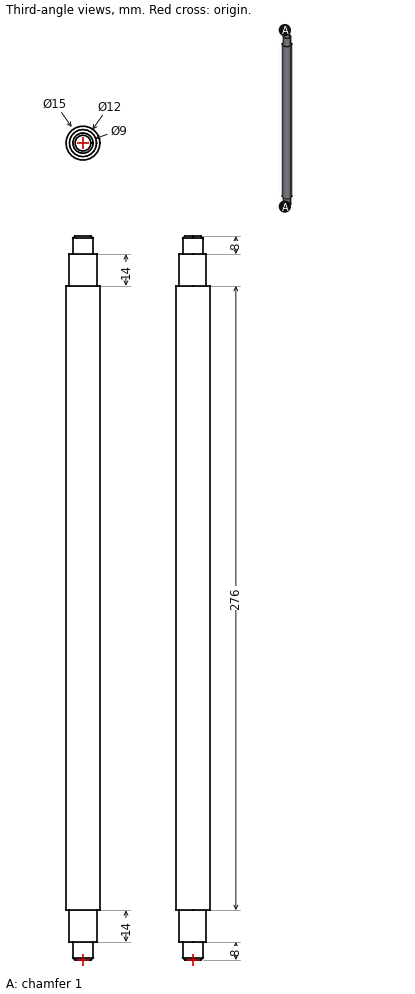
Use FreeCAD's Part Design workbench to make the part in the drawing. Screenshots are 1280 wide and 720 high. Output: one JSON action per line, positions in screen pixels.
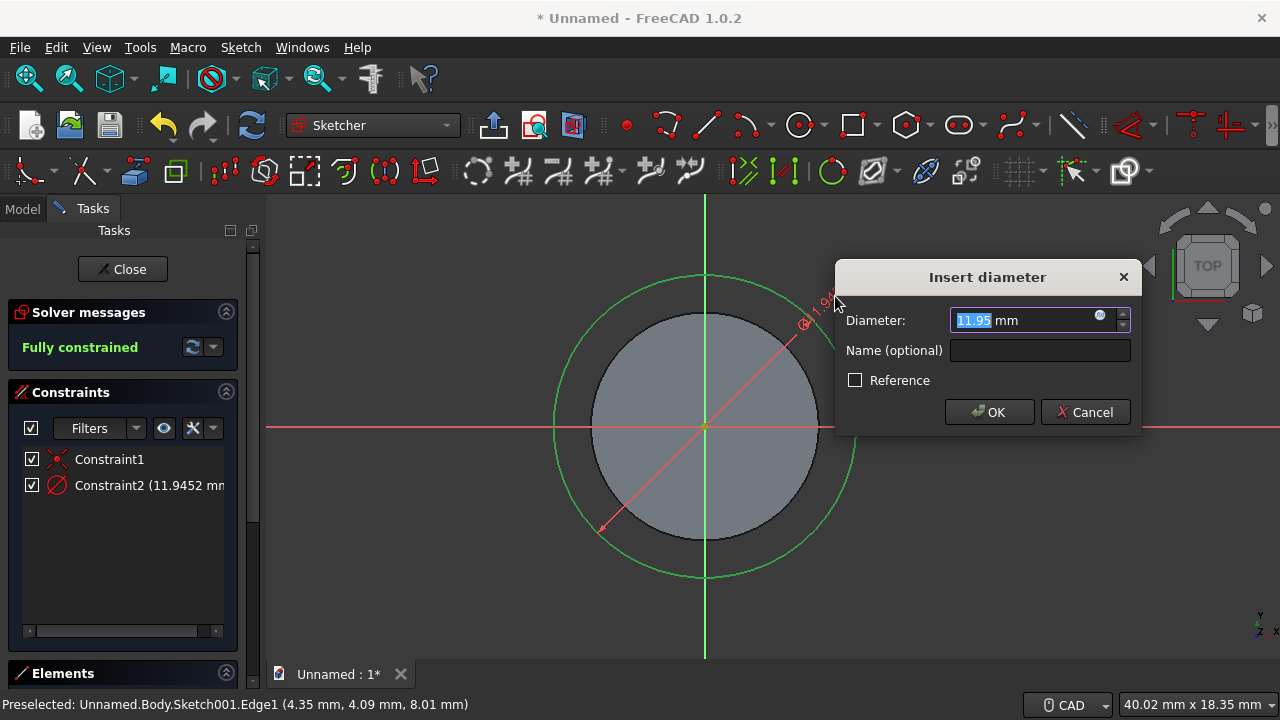
{"action": "type", "text": "12"}
{"action": "key", "text": "Return"}
{"action": "key", "text": "Escape"}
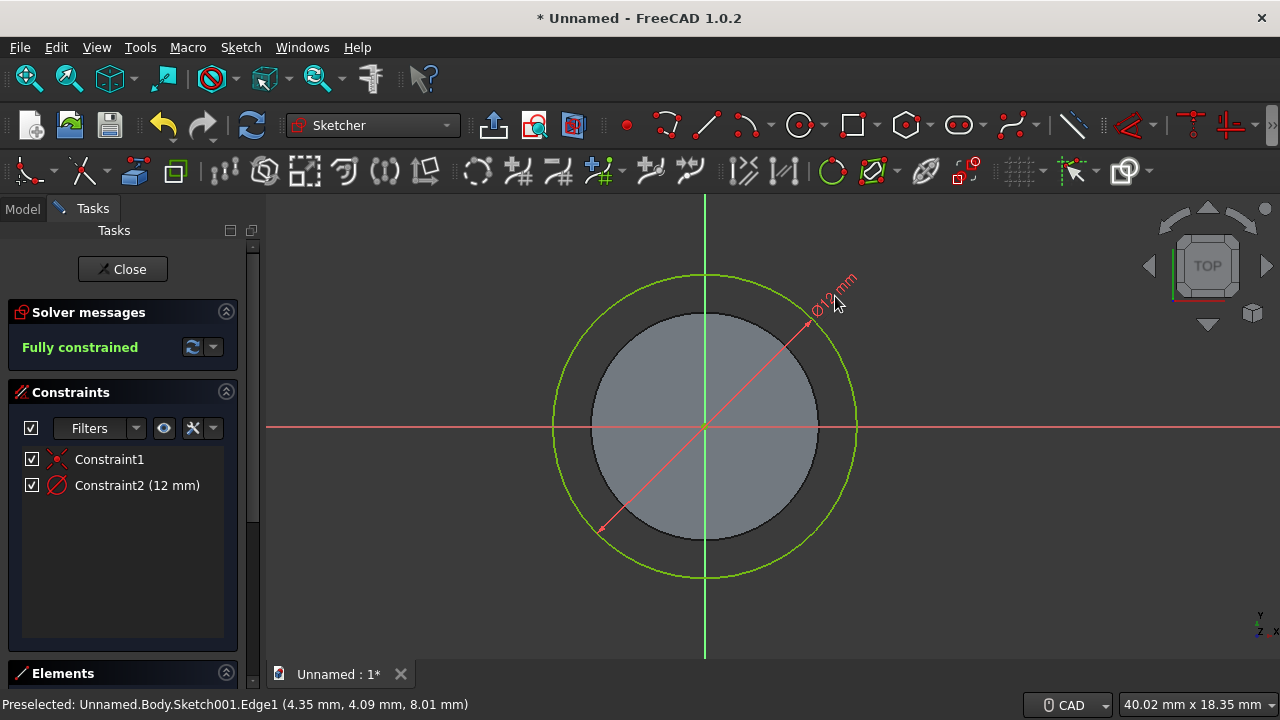
{"action": "left_click", "coordinate": [123, 269]}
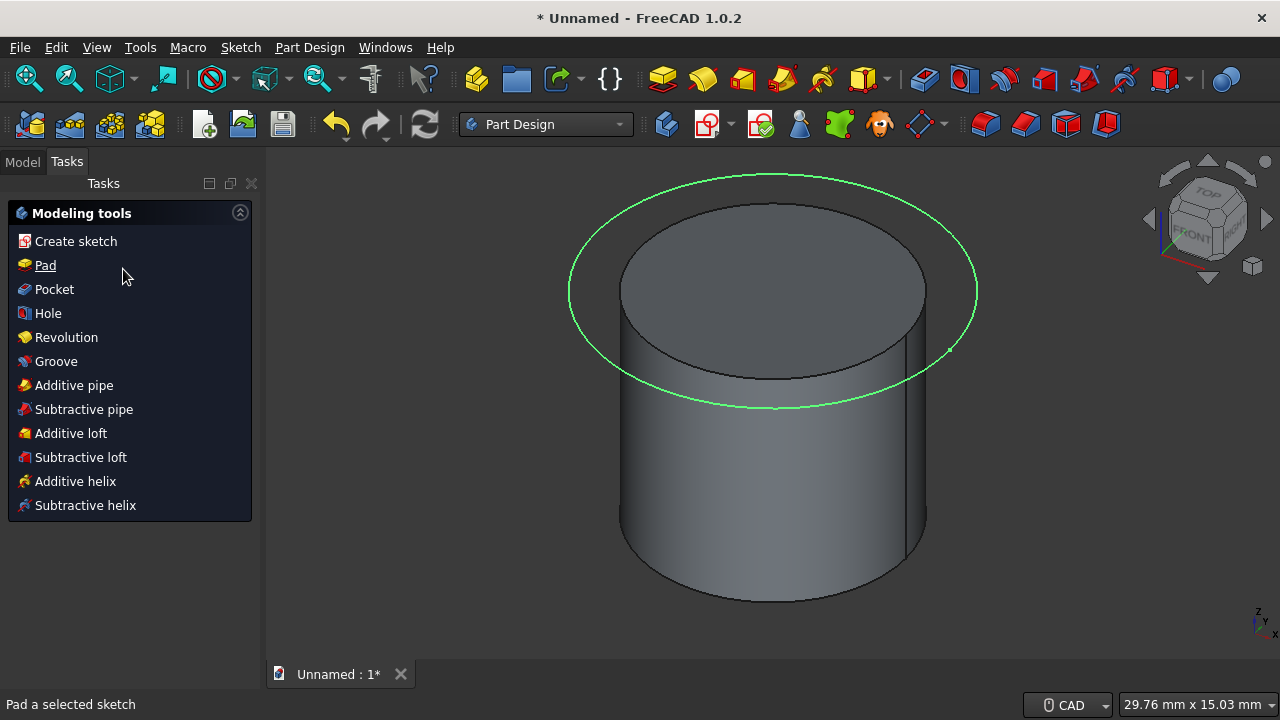
{"action": "left_click", "coordinate": [664, 80]}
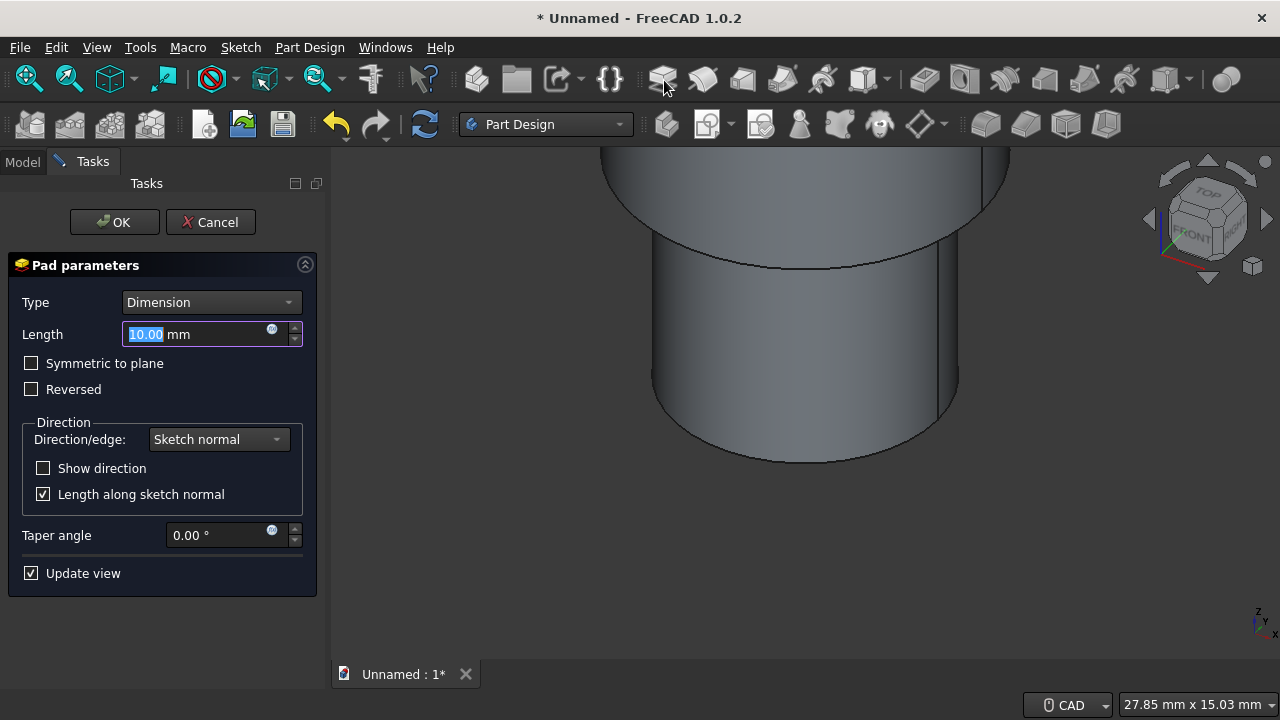
{"action": "type", "text": "14"}
{"action": "key", "text": "Tab"}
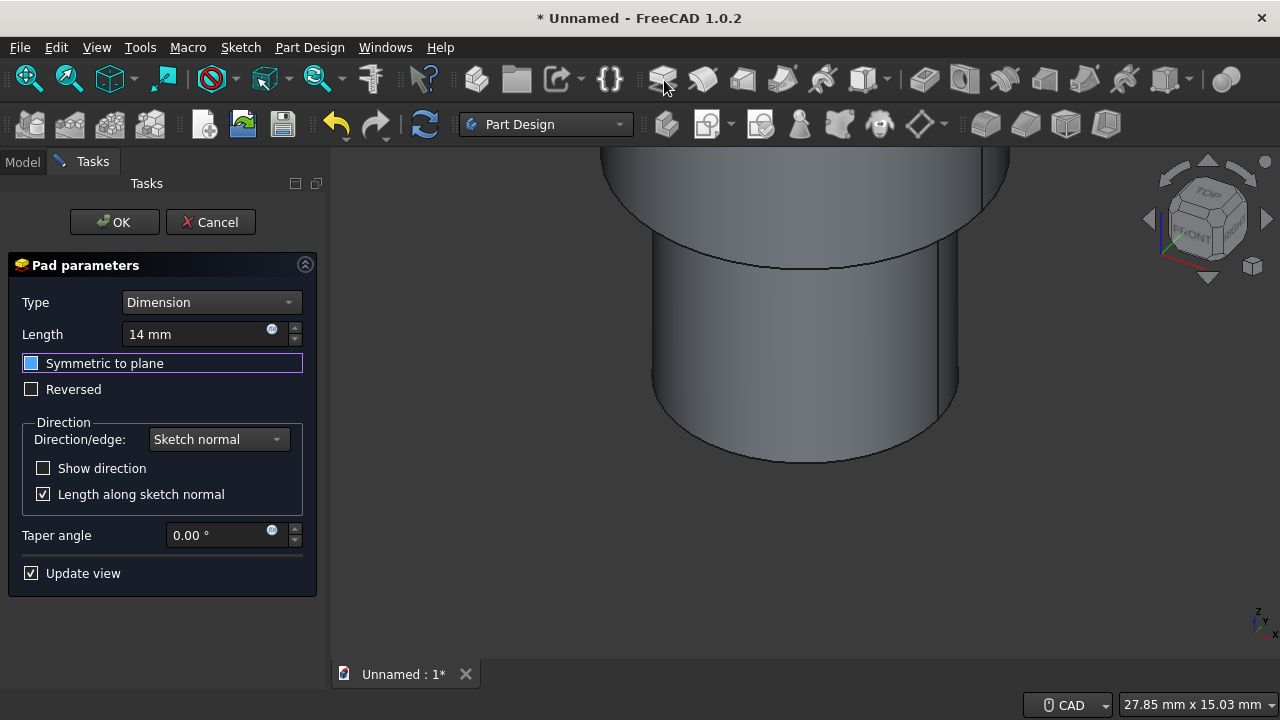
{"action": "left_click", "coordinate": [115, 222]}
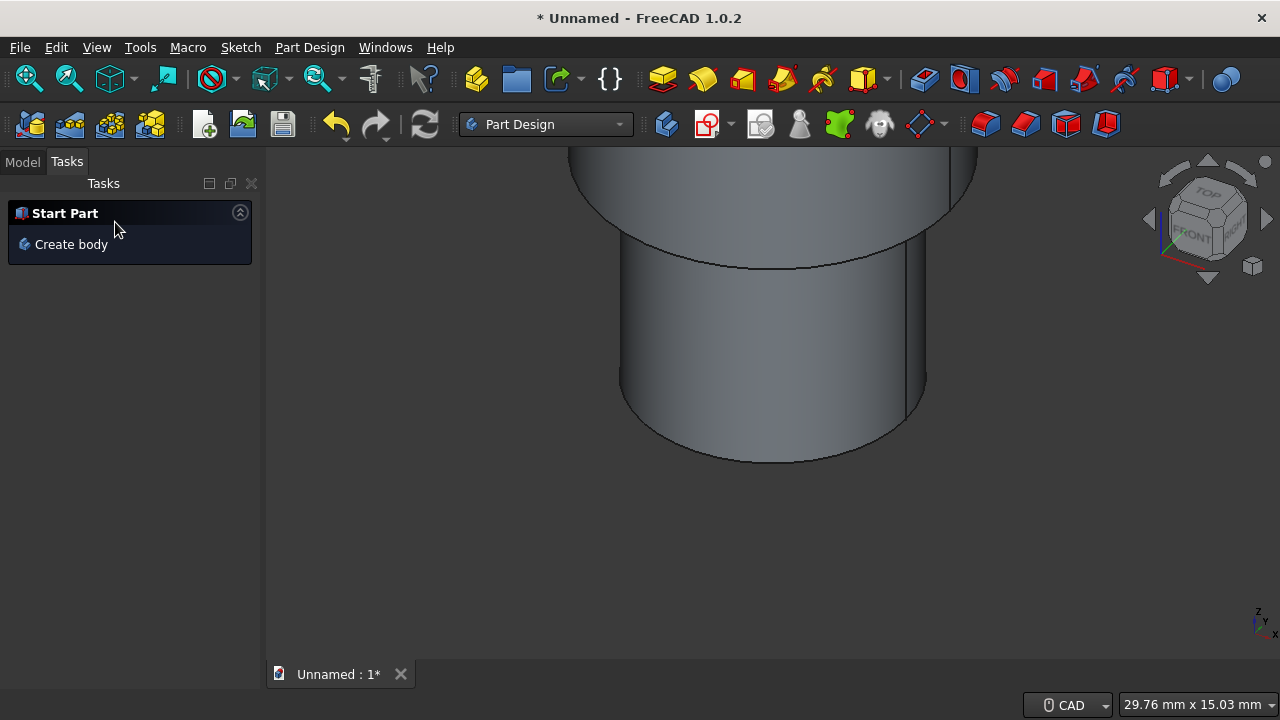
{"action": "left_click", "coordinate": [30, 80]}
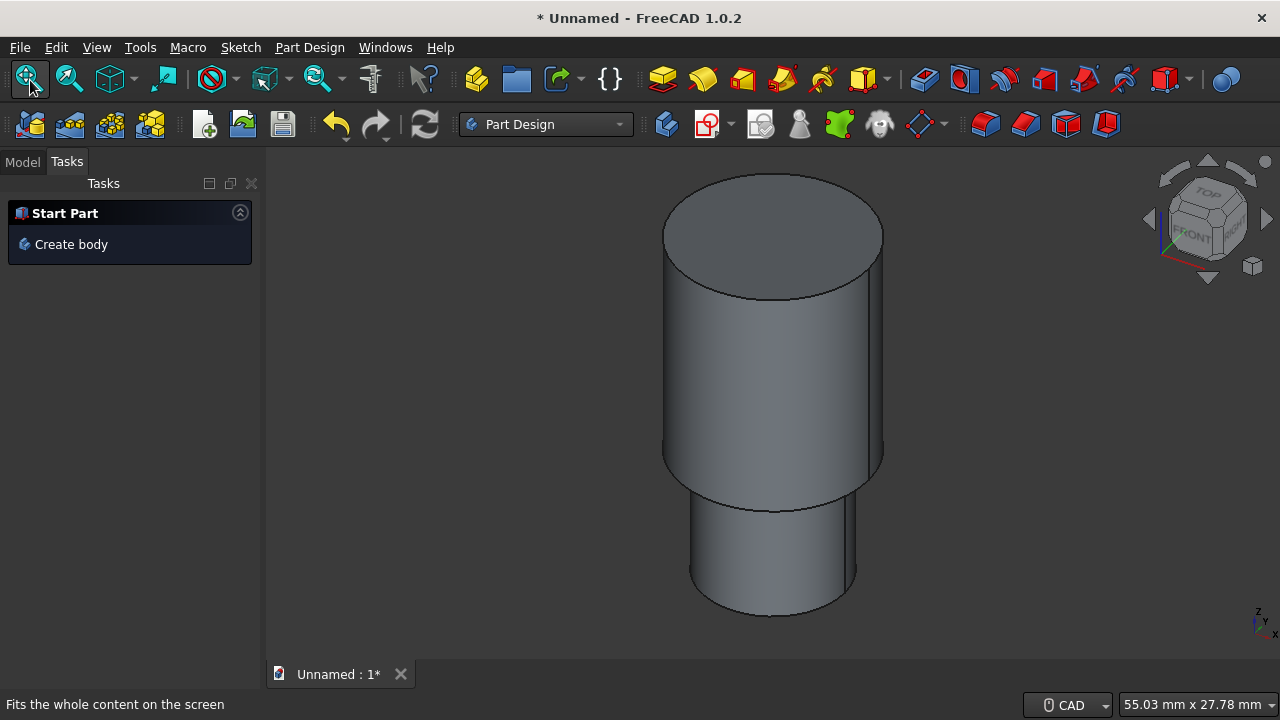
{"action": "left_click", "coordinate": [773, 236]}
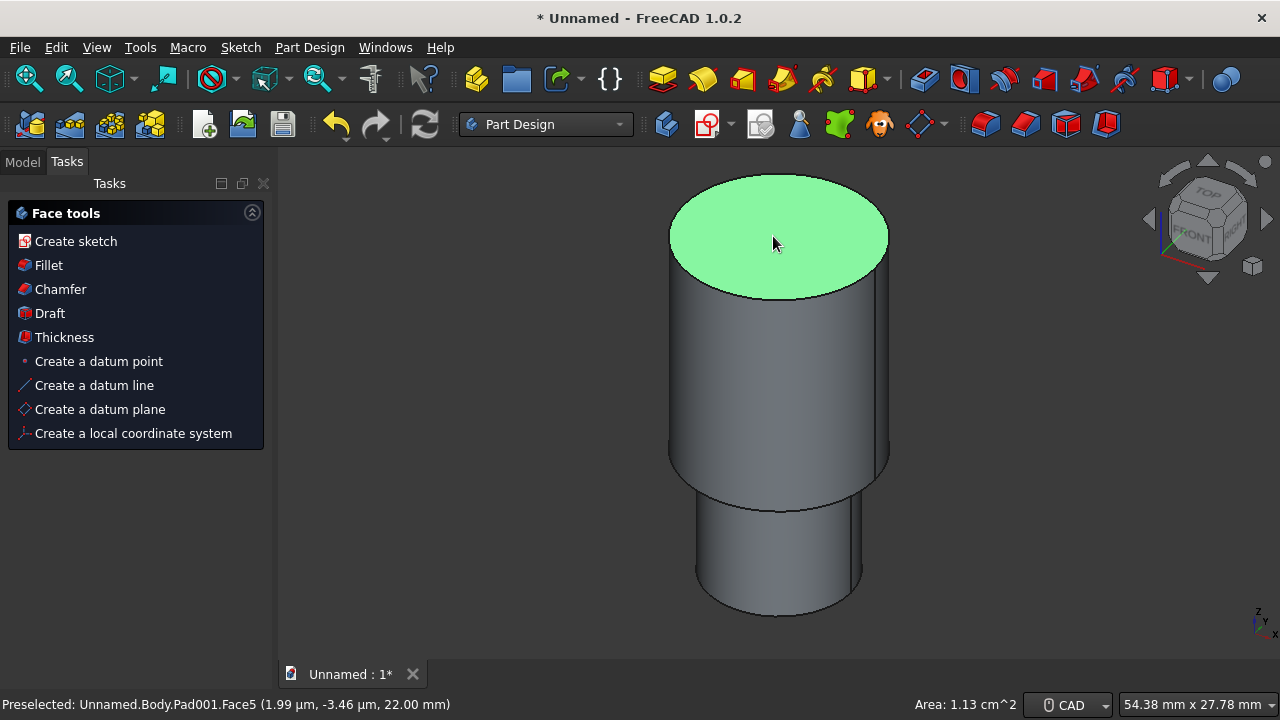
{"action": "left_click", "coordinate": [708, 124]}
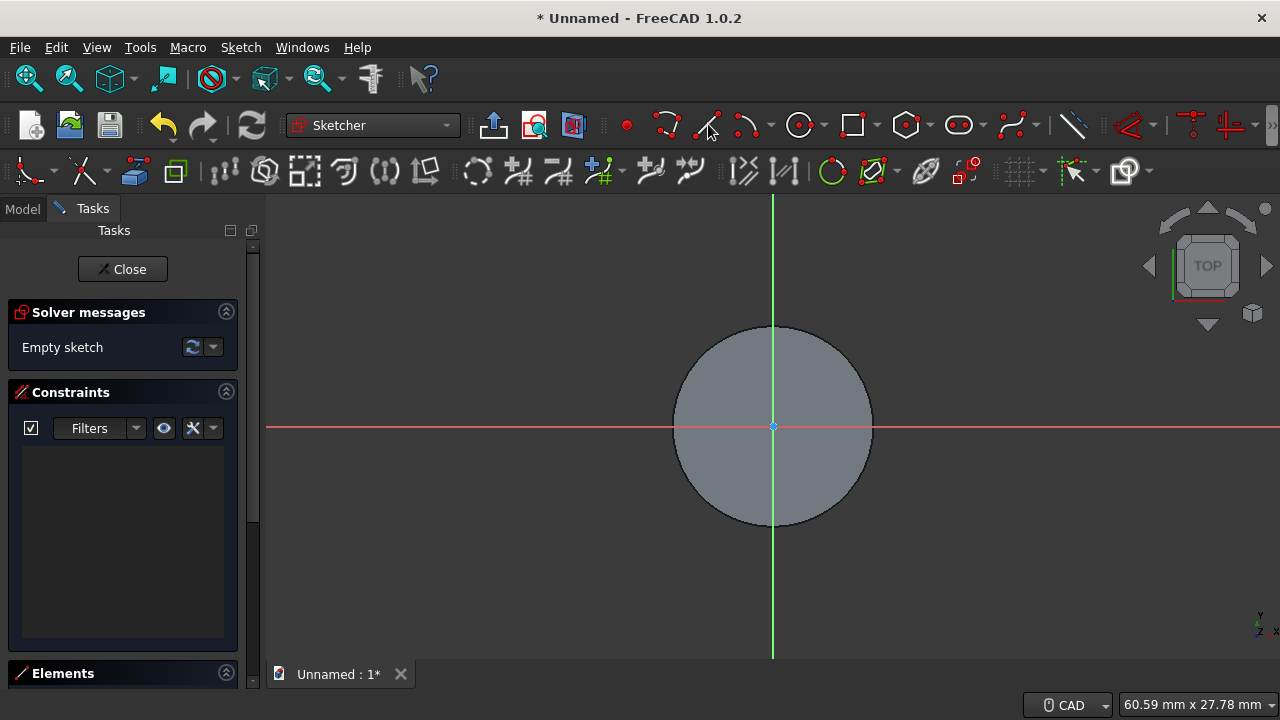
{"action": "key", "text": "g c"}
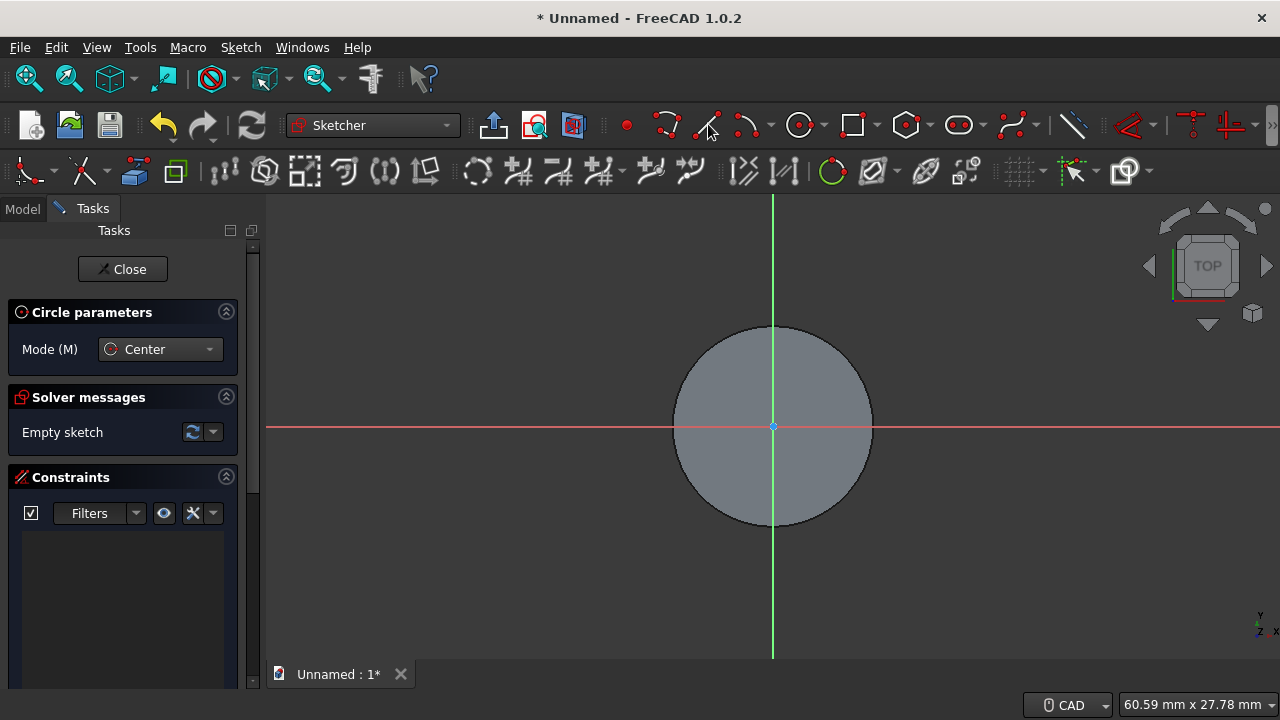
{"action": "left_click", "coordinate": [773, 426]}
{"action": "left_click", "coordinate": [862, 338]}
{"action": "key", "text": "Escape"}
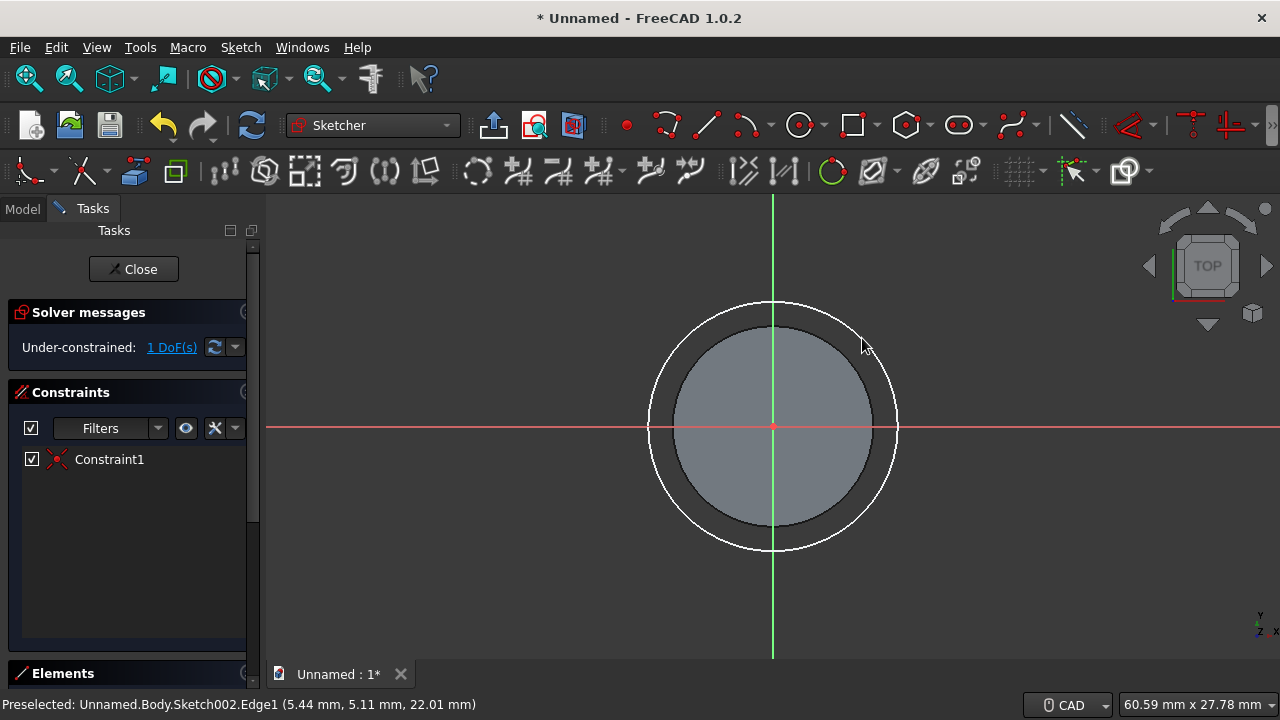
{"action": "left_click", "coordinate": [1128, 126]}